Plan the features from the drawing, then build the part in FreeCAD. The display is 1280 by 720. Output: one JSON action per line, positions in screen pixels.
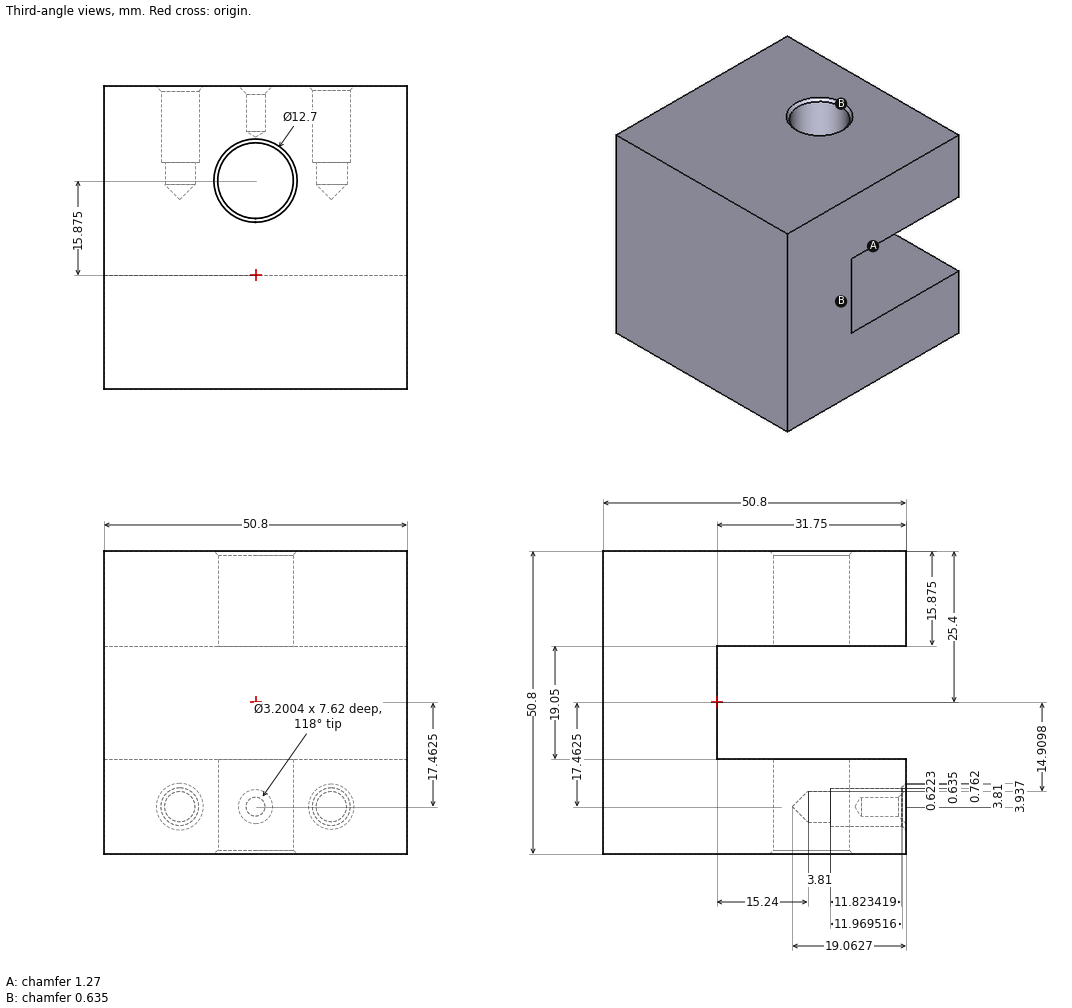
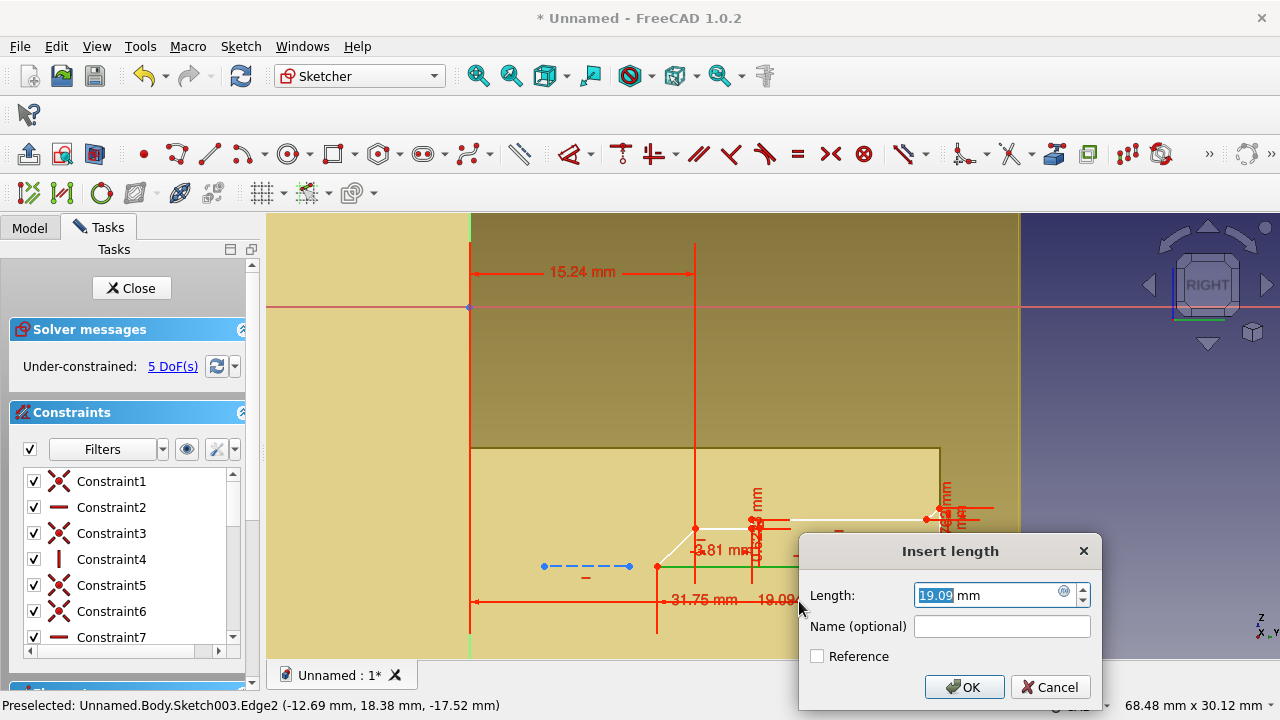
{"action": "type", "text": "19.0627"}
{"action": "key", "text": "Return"}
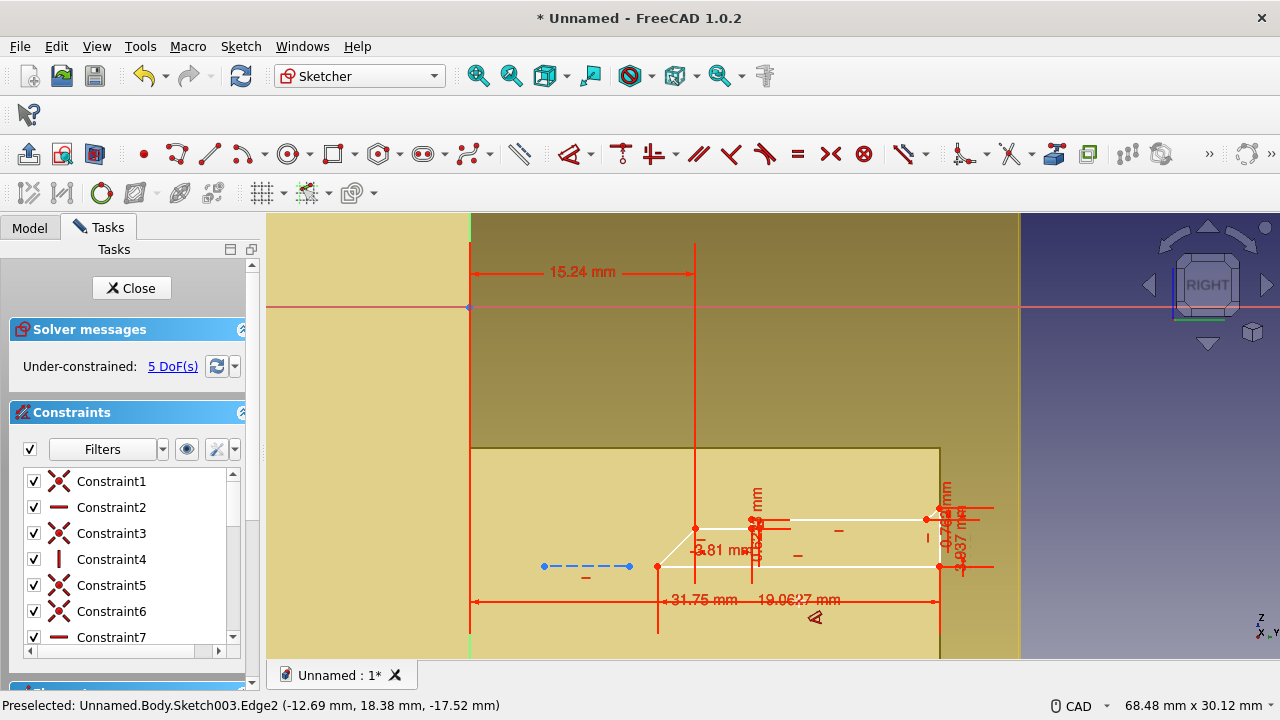
{"action": "left_click", "coordinate": [695, 529]}
{"action": "left_click", "coordinate": [436, 418]}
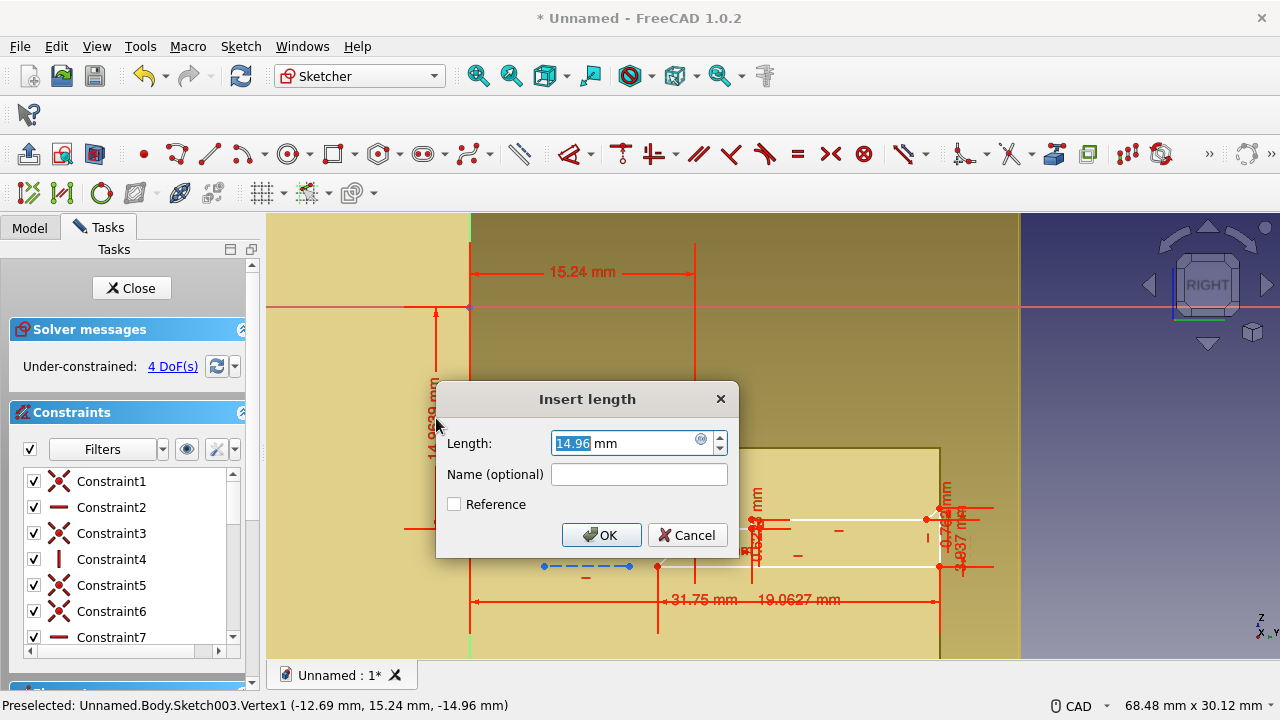
{"action": "type", "text": "14.9098"}
{"action": "key", "text": "Return"}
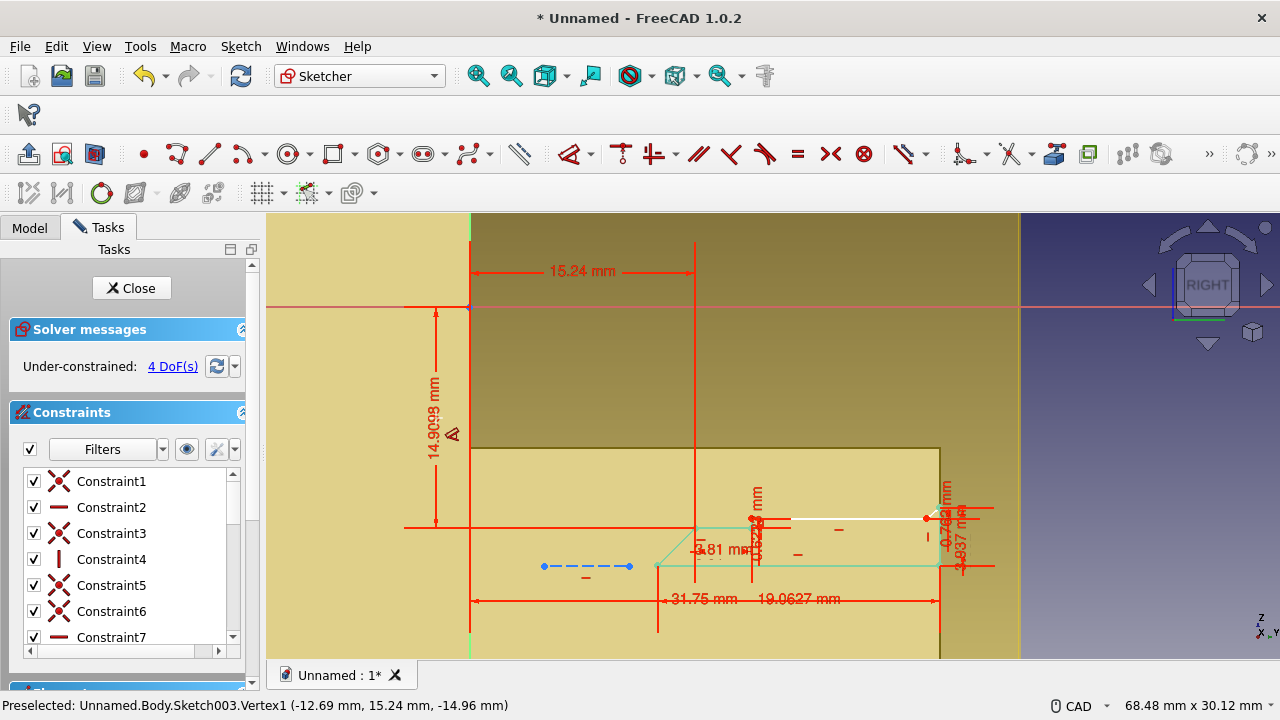
{"action": "left_click", "coordinate": [629, 566]}
{"action": "left_click", "coordinate": [436, 377]}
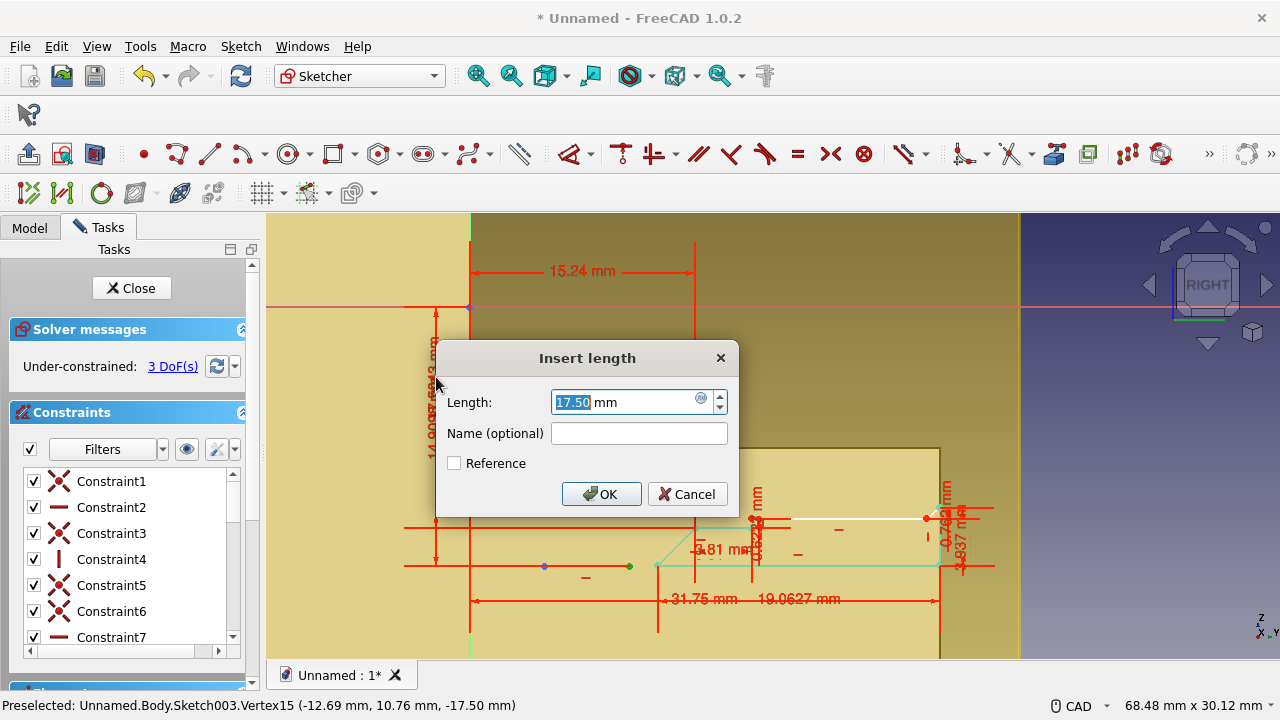
{"action": "type", "text": "17.4625"}
{"action": "key", "text": "Return"}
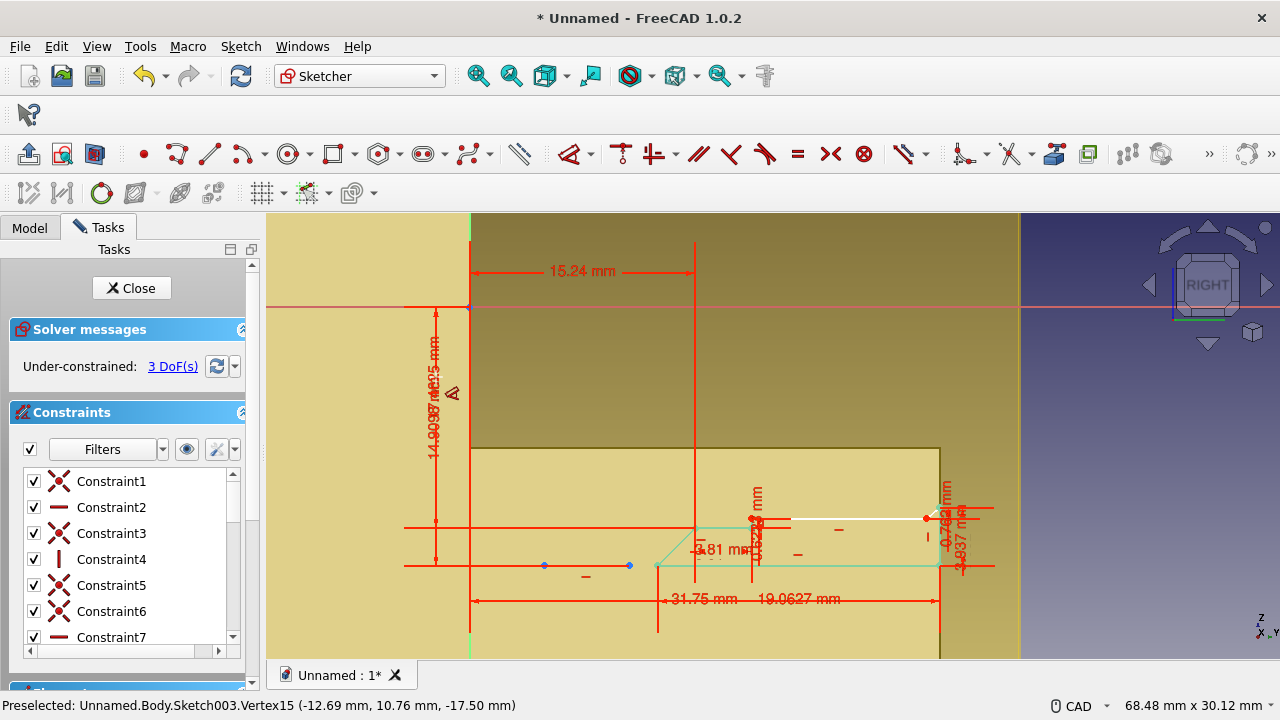
{"action": "left_click", "coordinate": [874, 519]}
{"action": "left_click", "coordinate": [839, 553]}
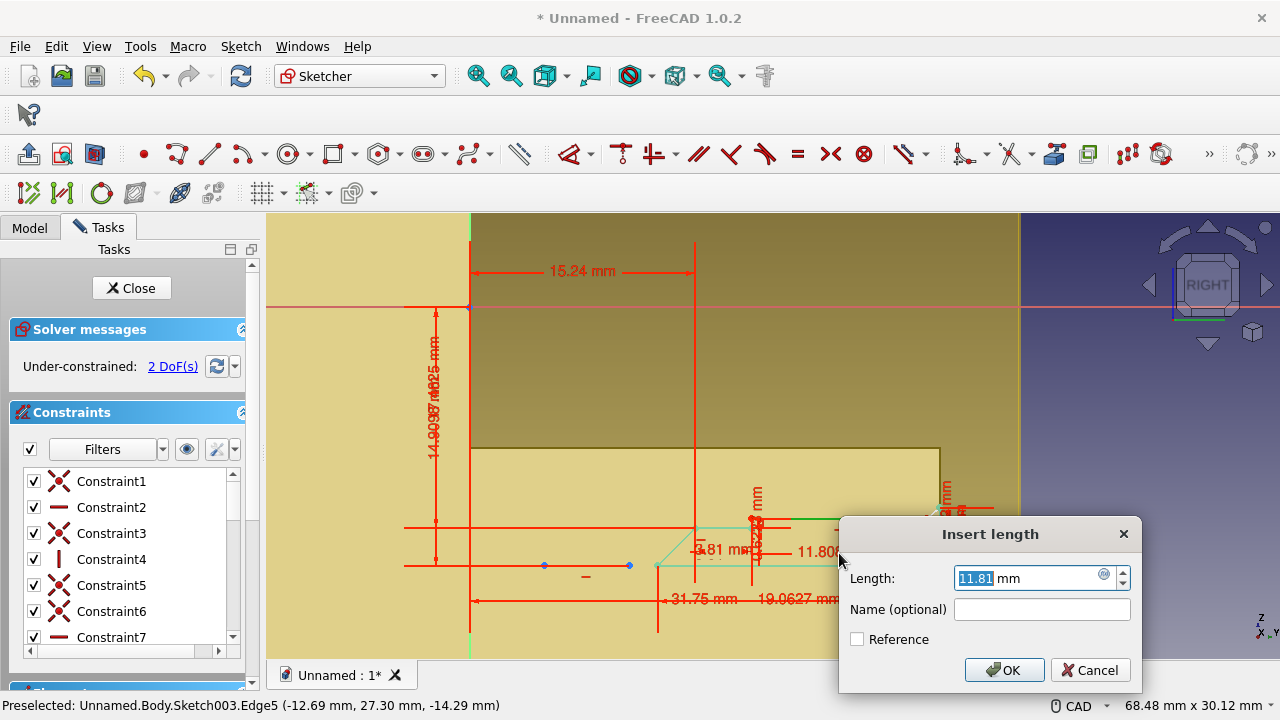
{"action": "type", "text": "11.823419"}
{"action": "key", "text": "Return"}
{"action": "key", "text": "Escape"}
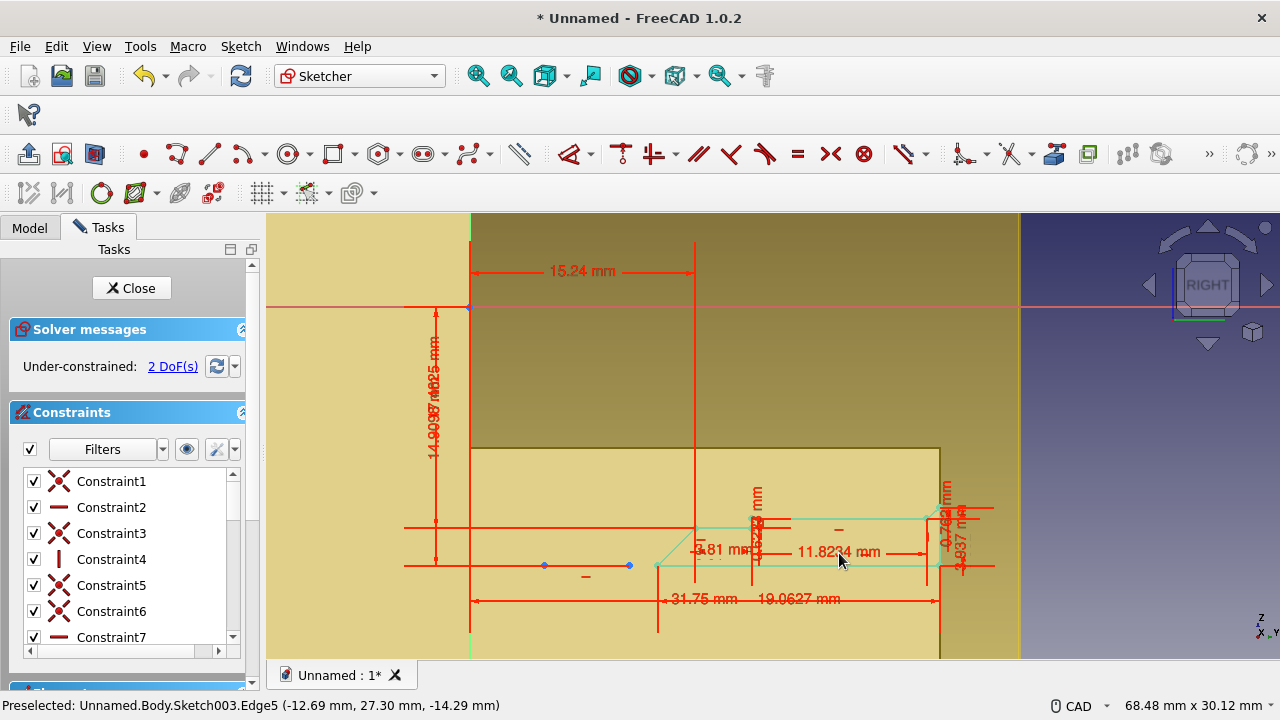
{"action": "left_click", "coordinate": [132, 288]}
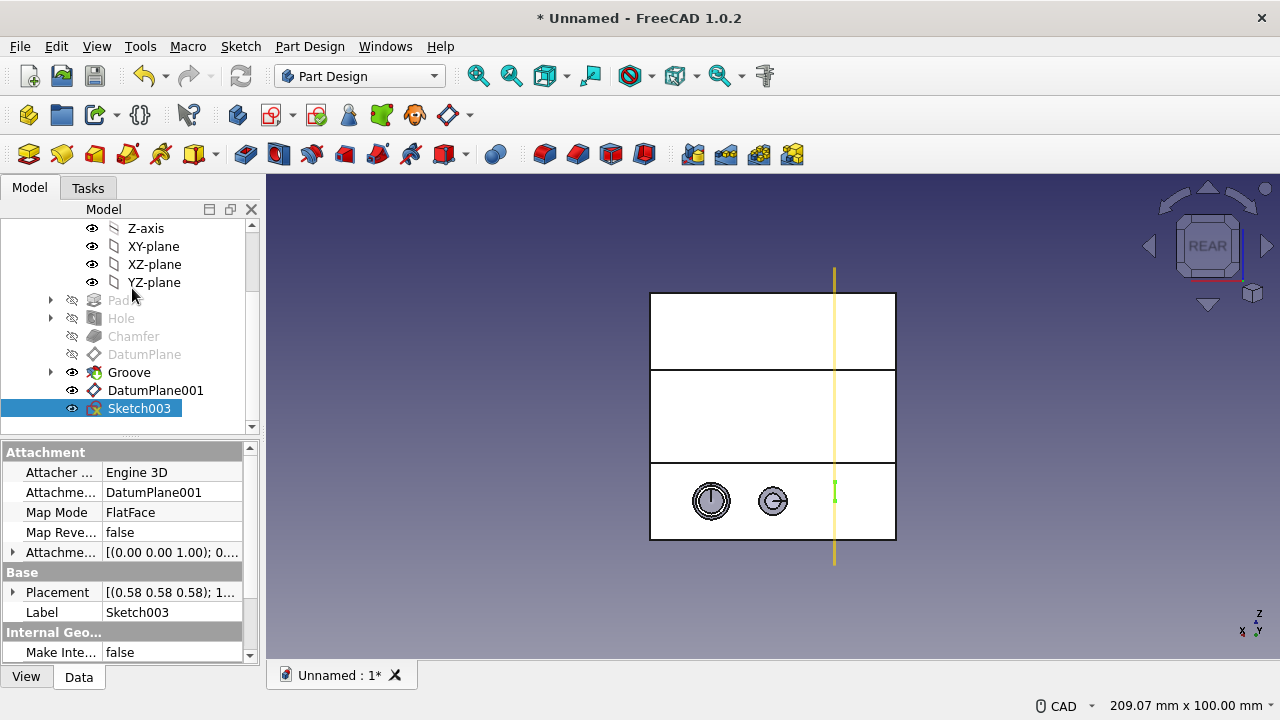
{"action": "left_click", "coordinate": [312, 154]}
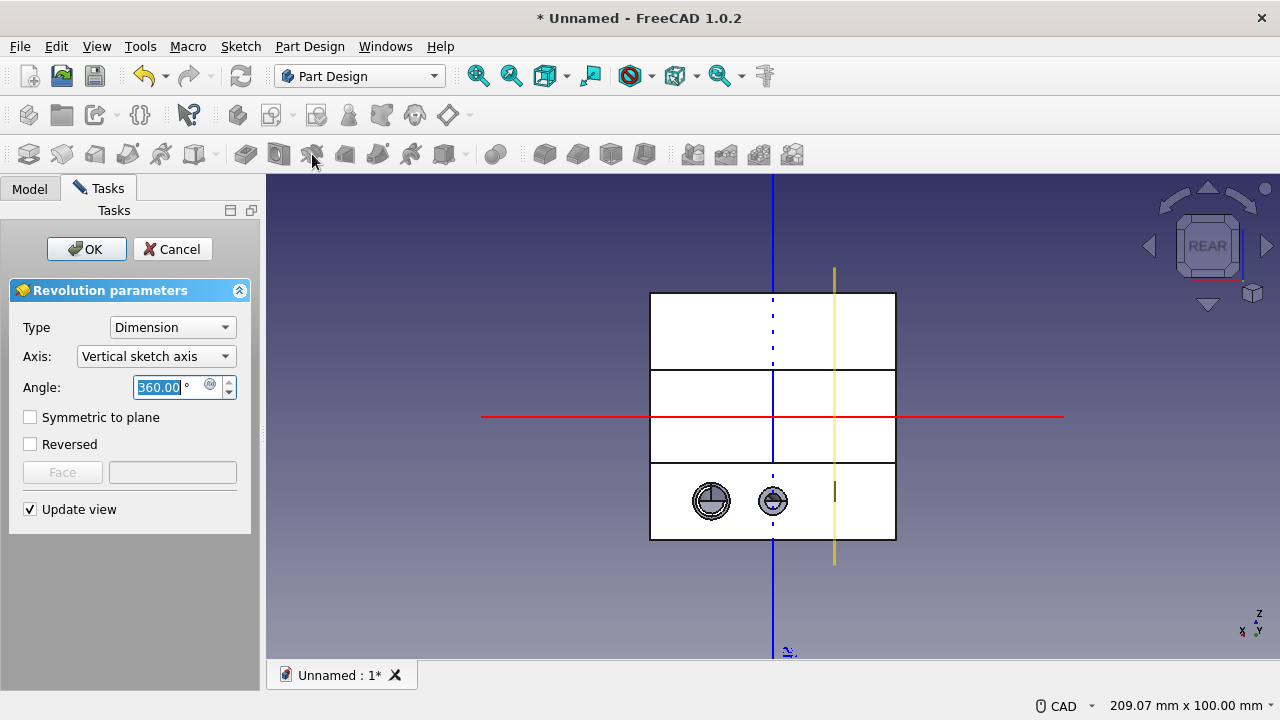
{"action": "left_click", "coordinate": [157, 356]}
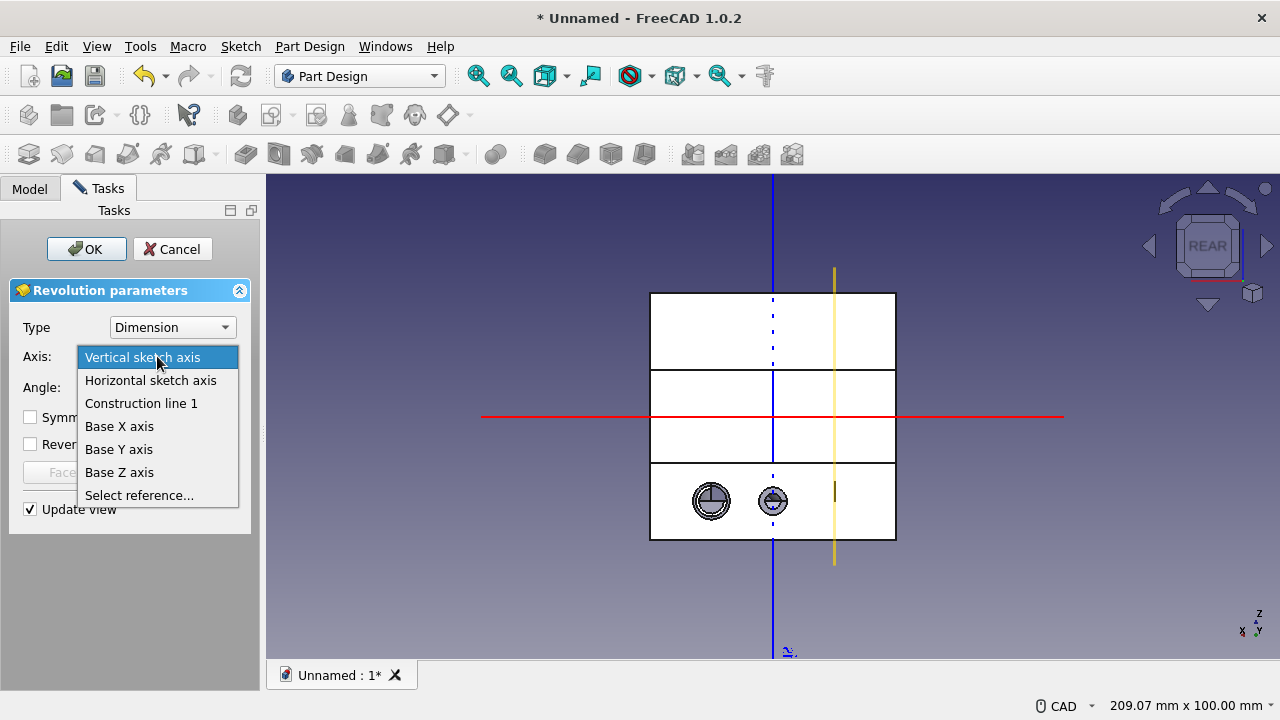
{"action": "left_click", "coordinate": [156, 404]}